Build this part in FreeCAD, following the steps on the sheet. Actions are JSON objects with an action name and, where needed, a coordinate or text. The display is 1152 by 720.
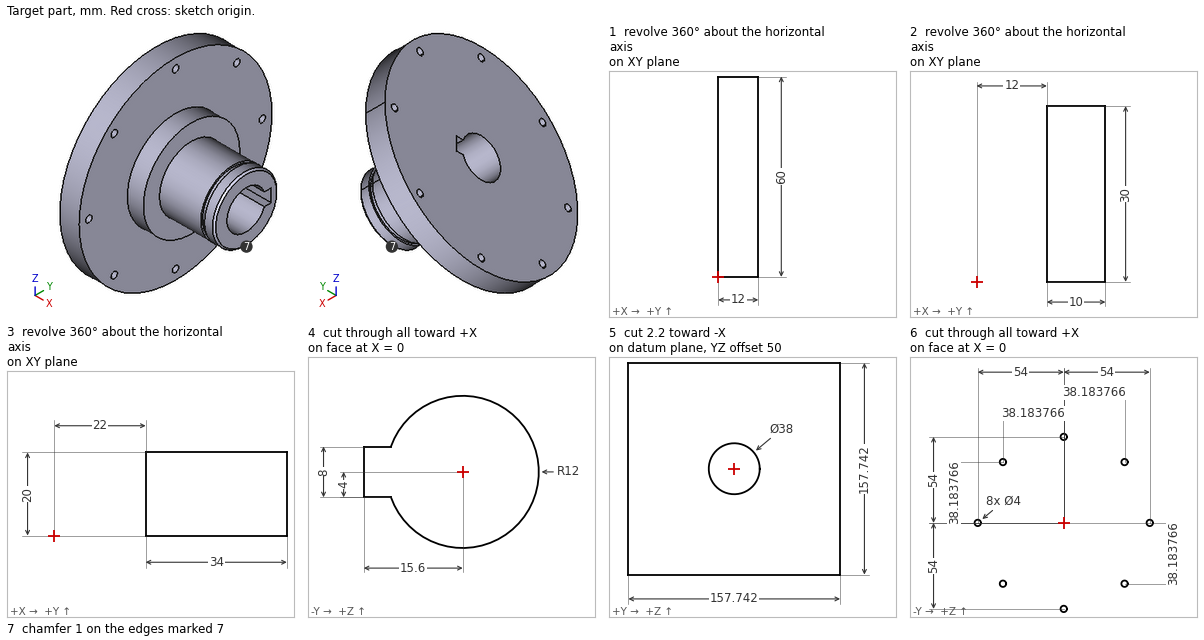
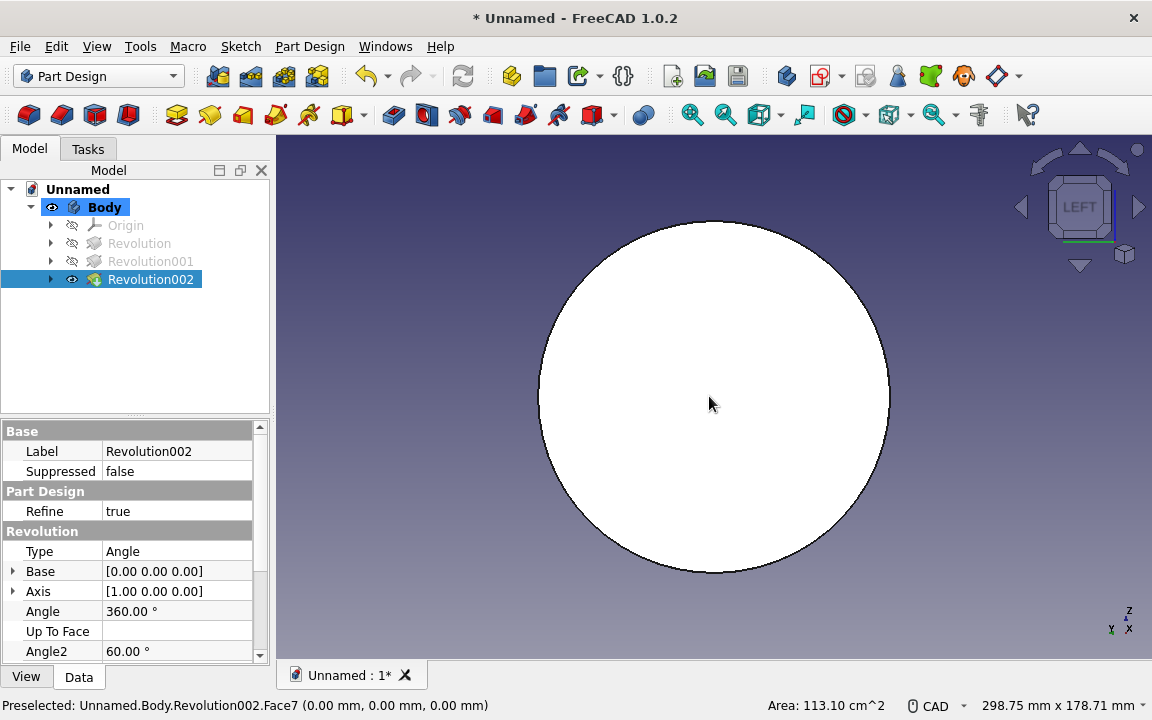
{"action": "left_click", "coordinate": [820, 76]}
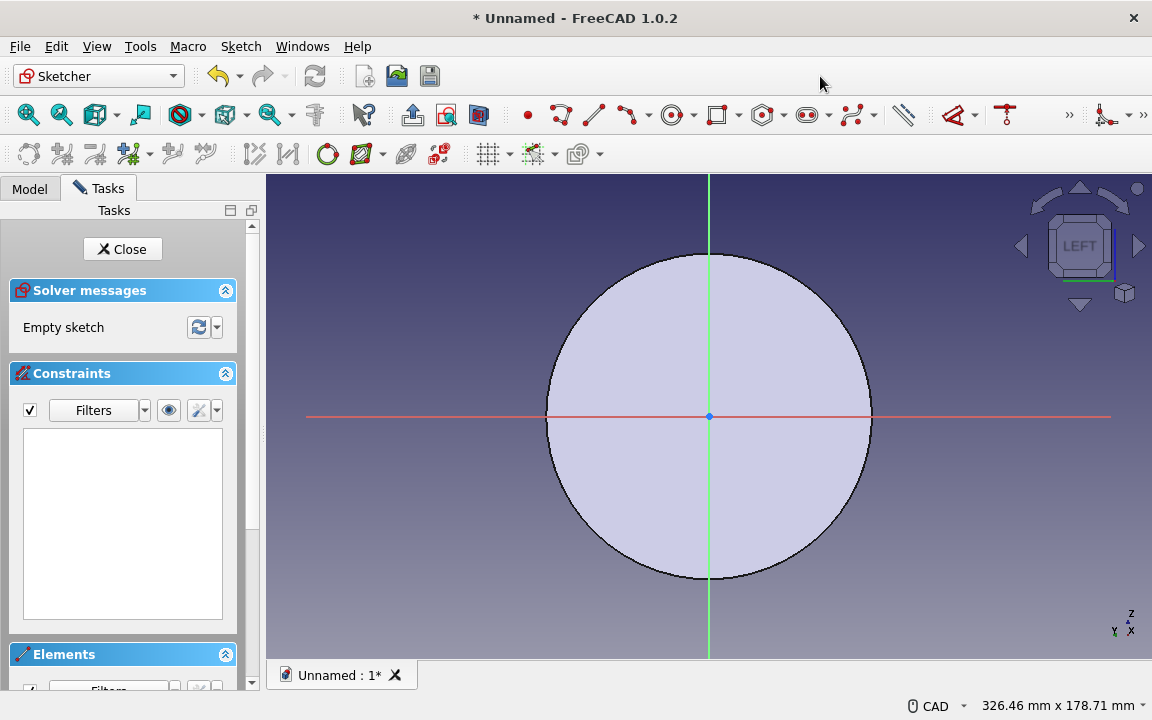
{"action": "scroll", "coordinate": [717, 416], "scroll_direction": "up", "scroll_amount": 9}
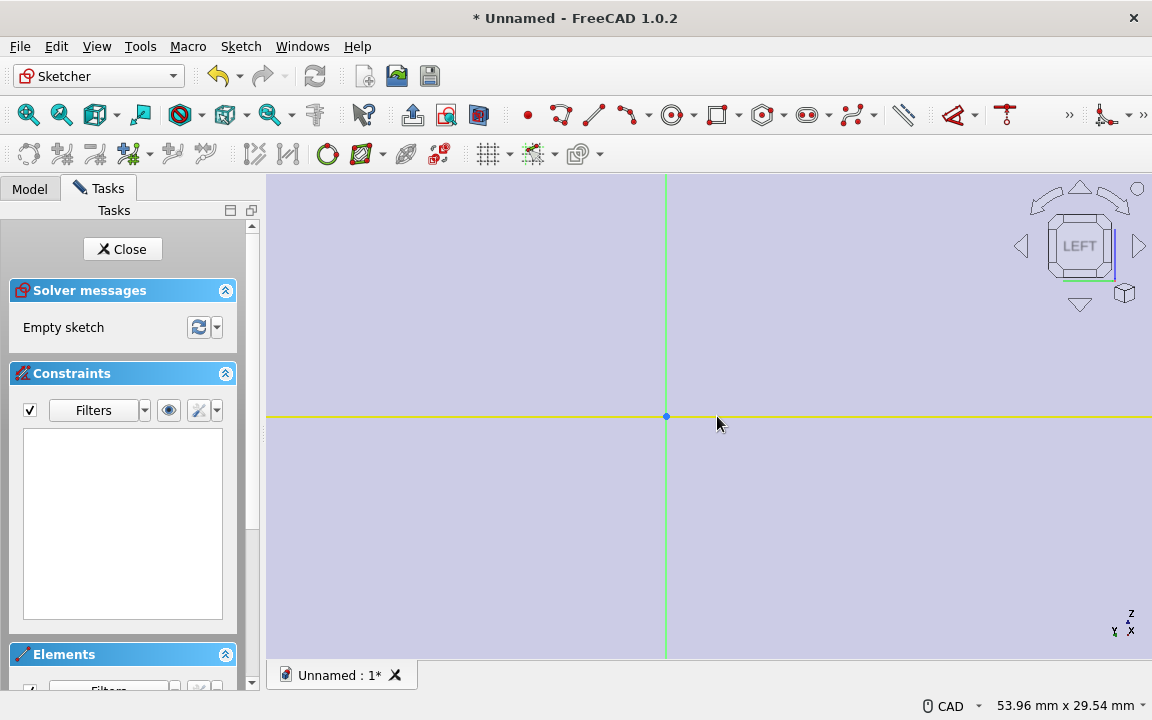
{"action": "left_click", "coordinate": [561, 116]}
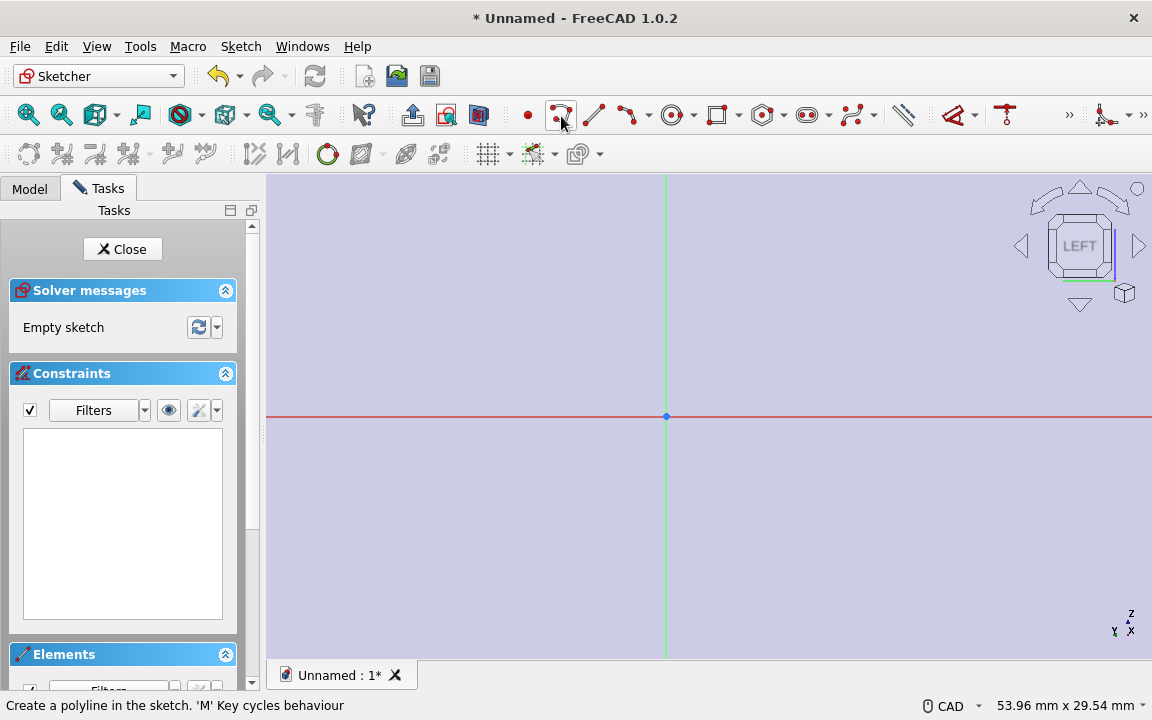
{"action": "left_click", "coordinate": [480, 482]}
{"action": "left_click", "coordinate": [410, 482]}
{"action": "left_click", "coordinate": [410, 351]}
{"action": "left_click", "coordinate": [480, 351]}
{"action": "right_click", "coordinate": [480, 351]}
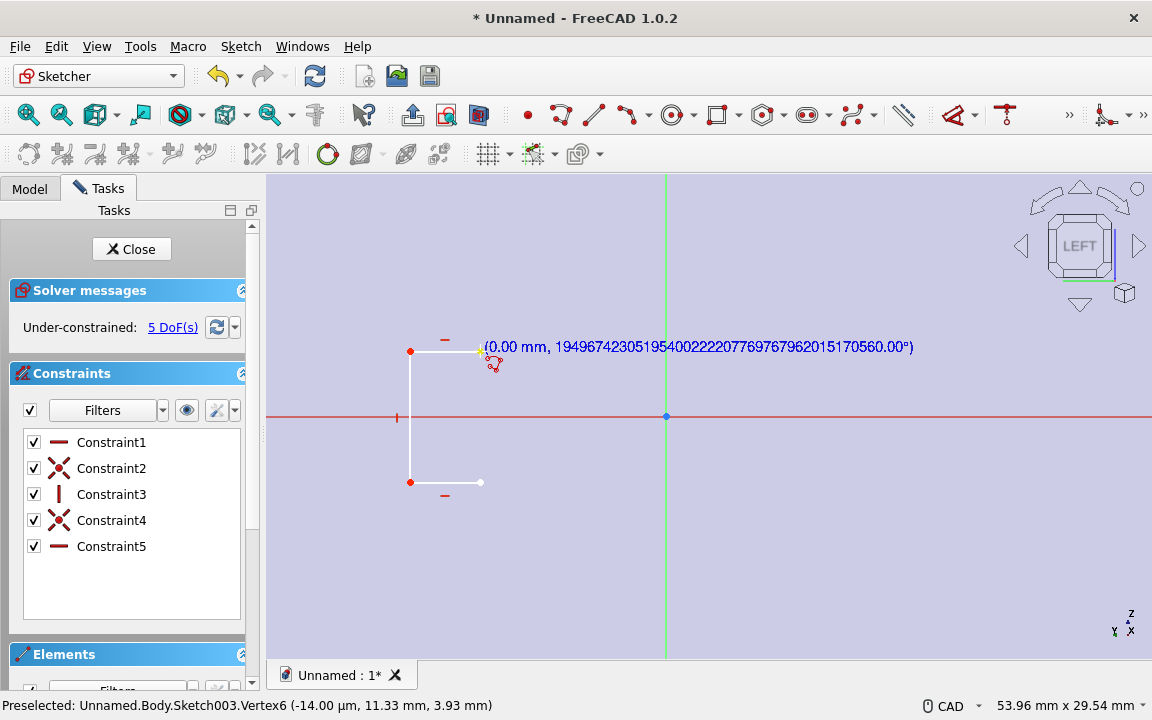
{"action": "left_click", "coordinate": [626, 116]}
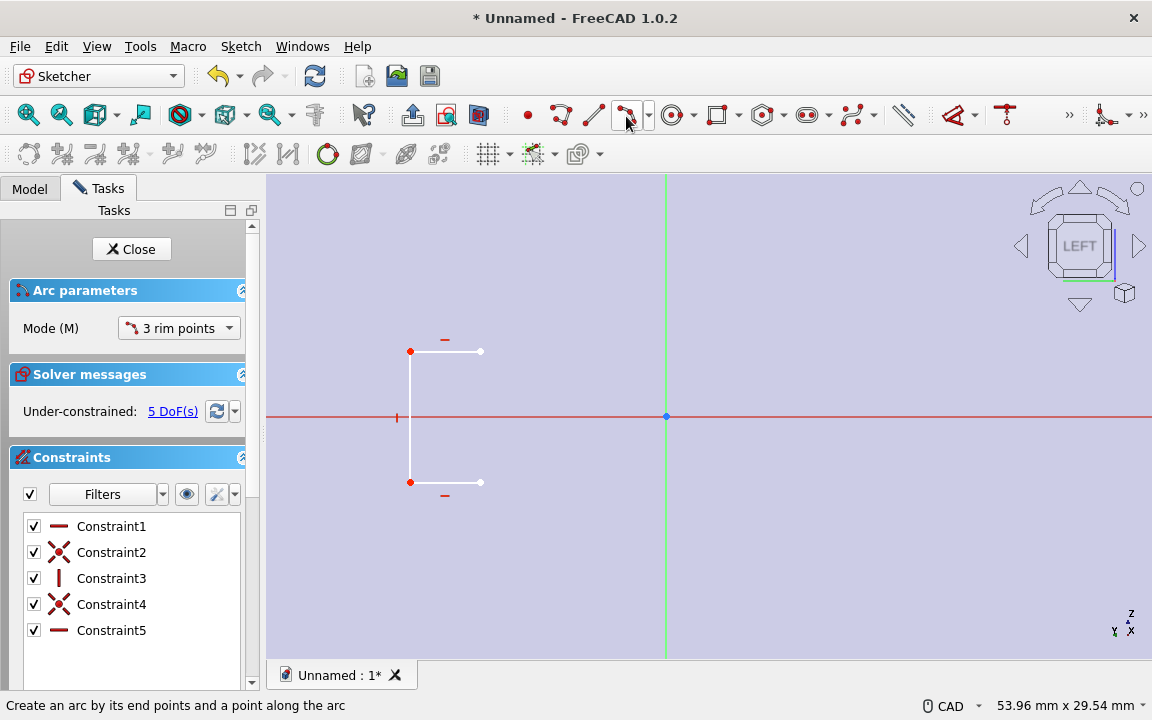
{"action": "left_click", "coordinate": [480, 352]}
{"action": "left_click", "coordinate": [480, 483]}
{"action": "left_click", "coordinate": [833, 521]}
{"action": "key", "text": "Escape"}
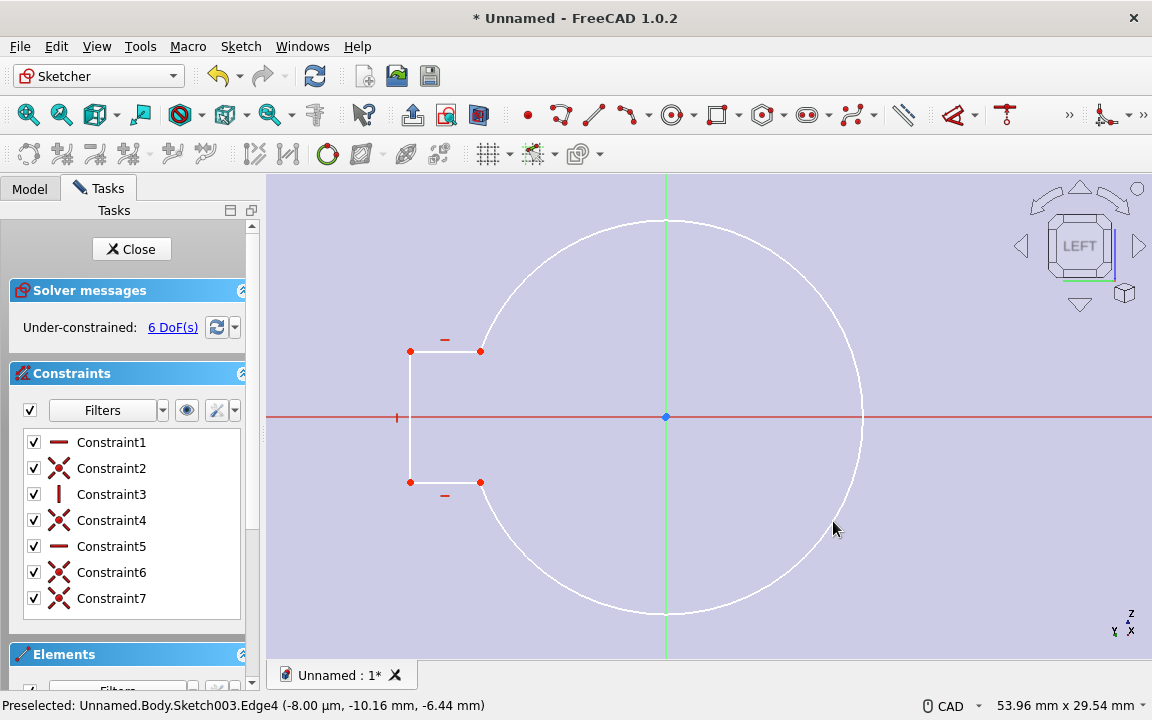
{"action": "left_click_drag", "start_coordinate": [656, 406], "coordinate": [676, 427]}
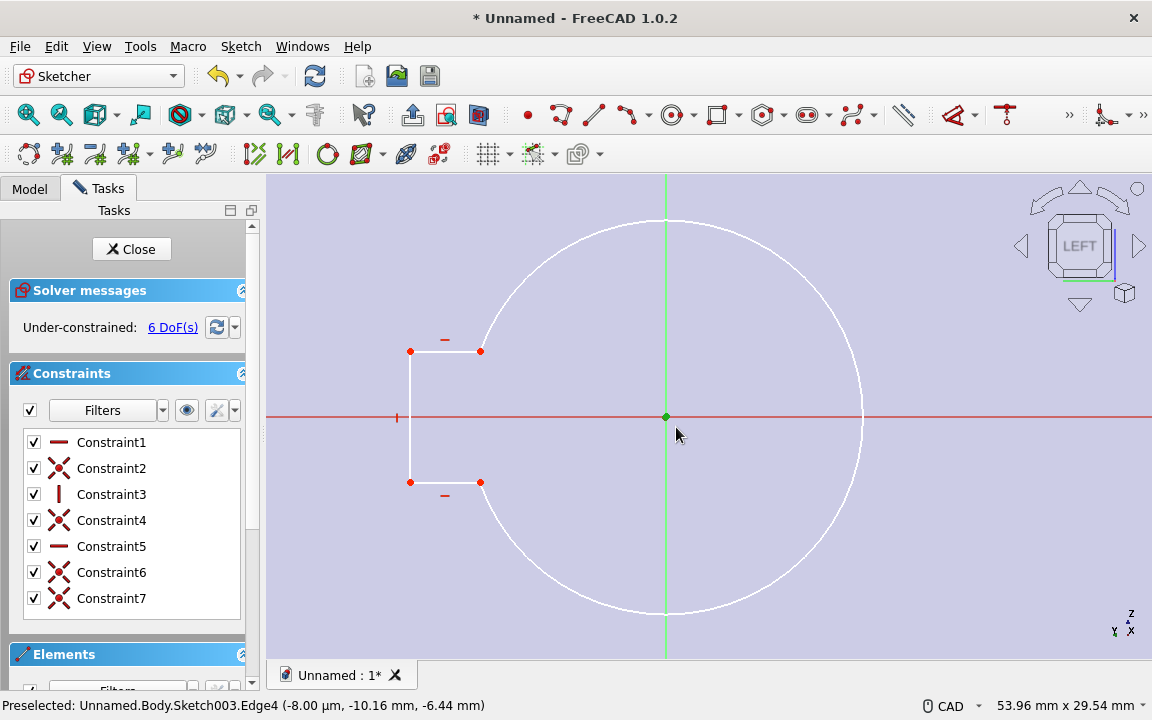
{"action": "left_click", "coordinate": [1005, 116]}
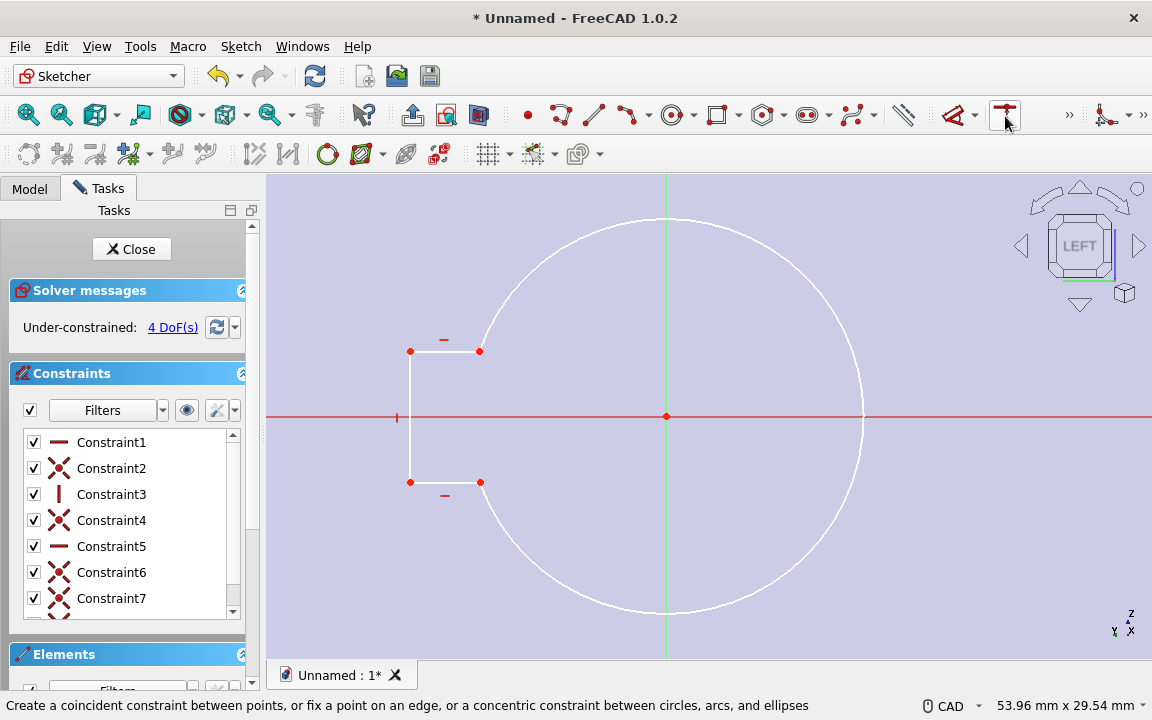
{"action": "left_click", "coordinate": [952, 116]}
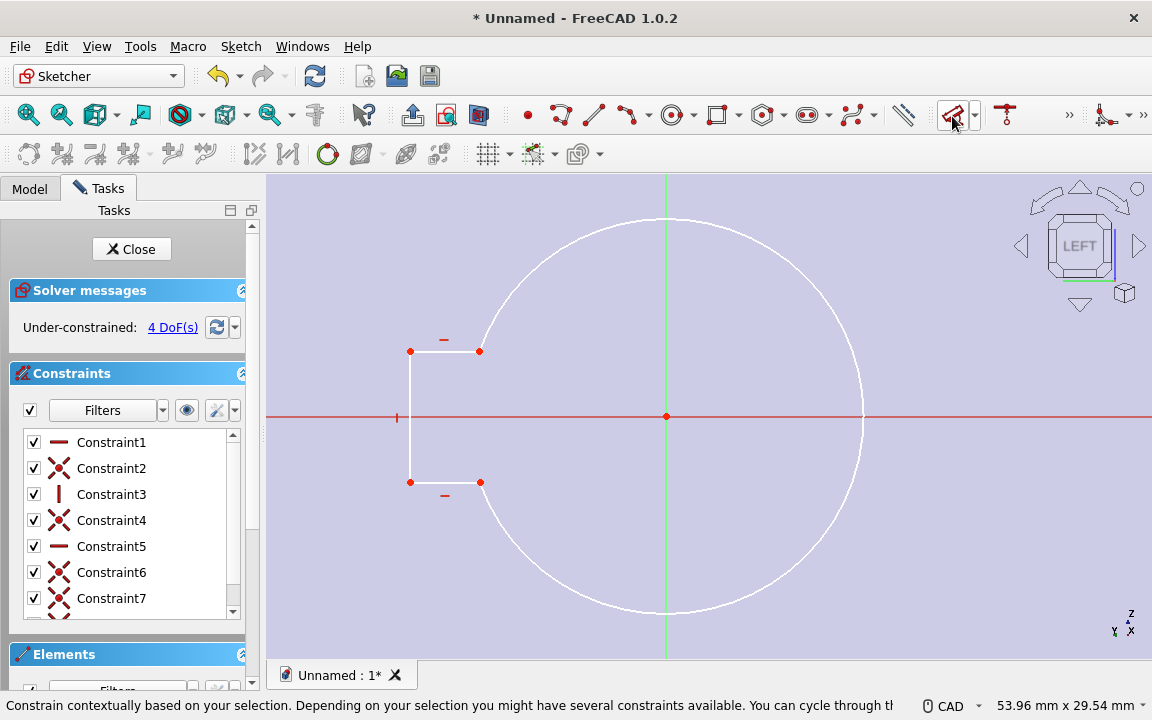
{"action": "left_click", "coordinate": [753, 594]}
{"action": "left_click", "coordinate": [767, 623]}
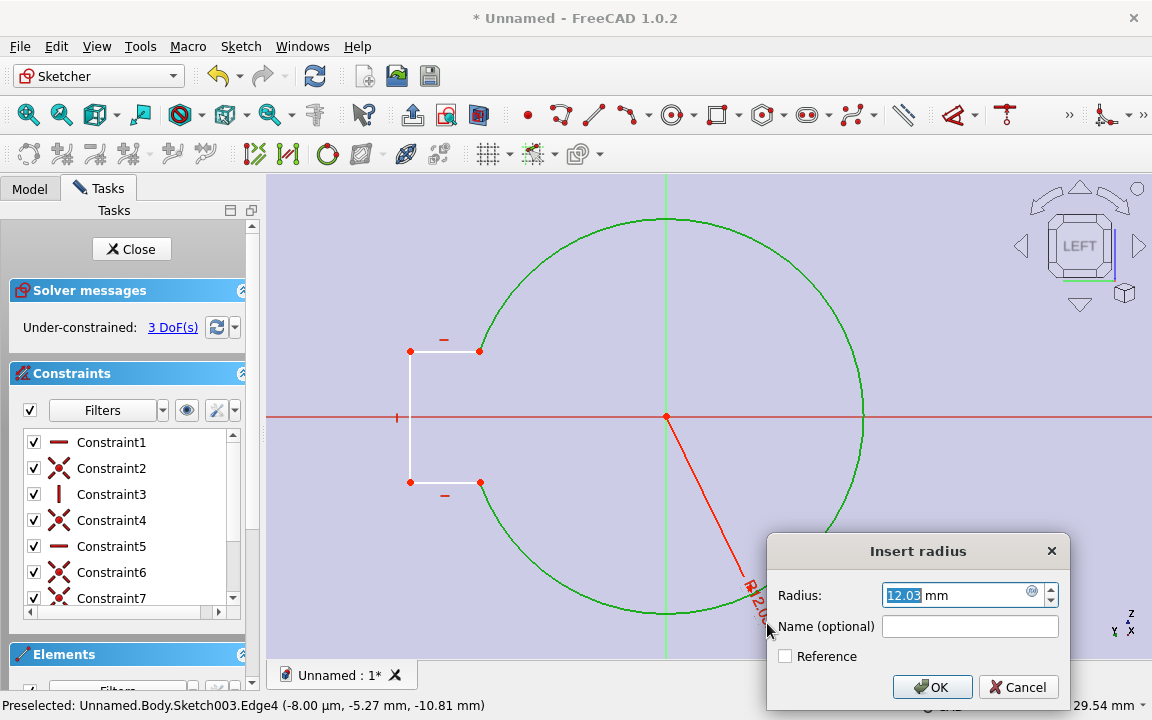
{"action": "type", "text": "12"}
{"action": "key", "text": "Return"}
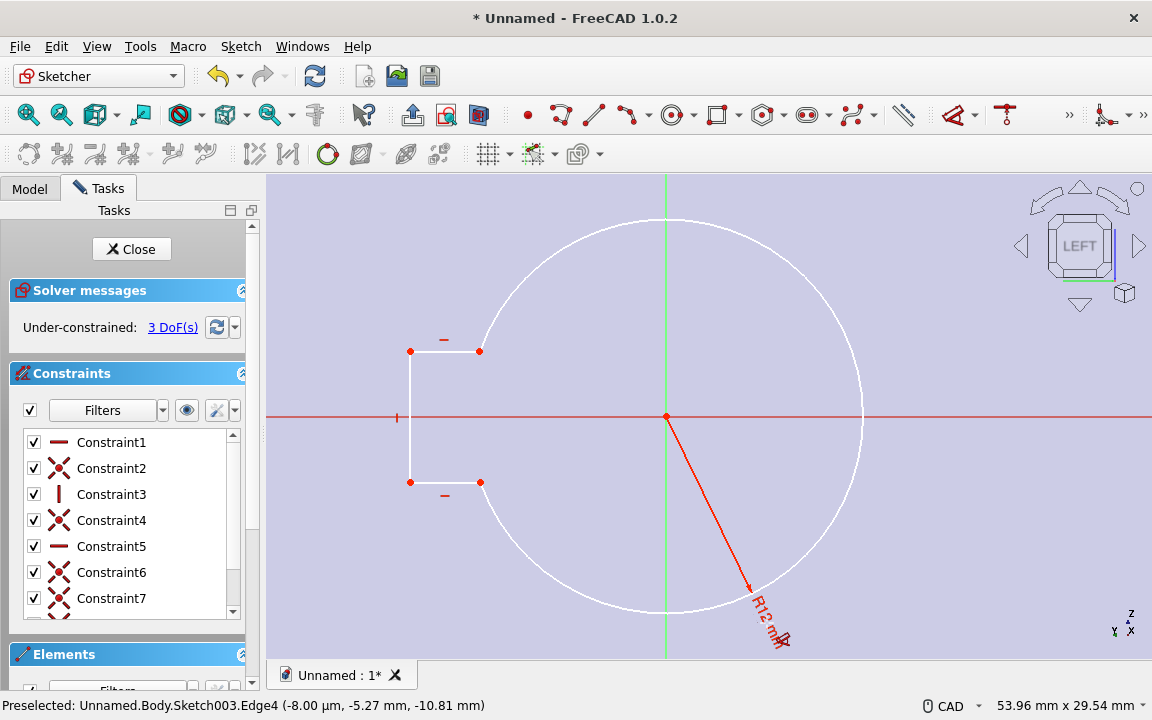
{"action": "left_click", "coordinate": [410, 444]}
{"action": "left_click", "coordinate": [376, 387]}